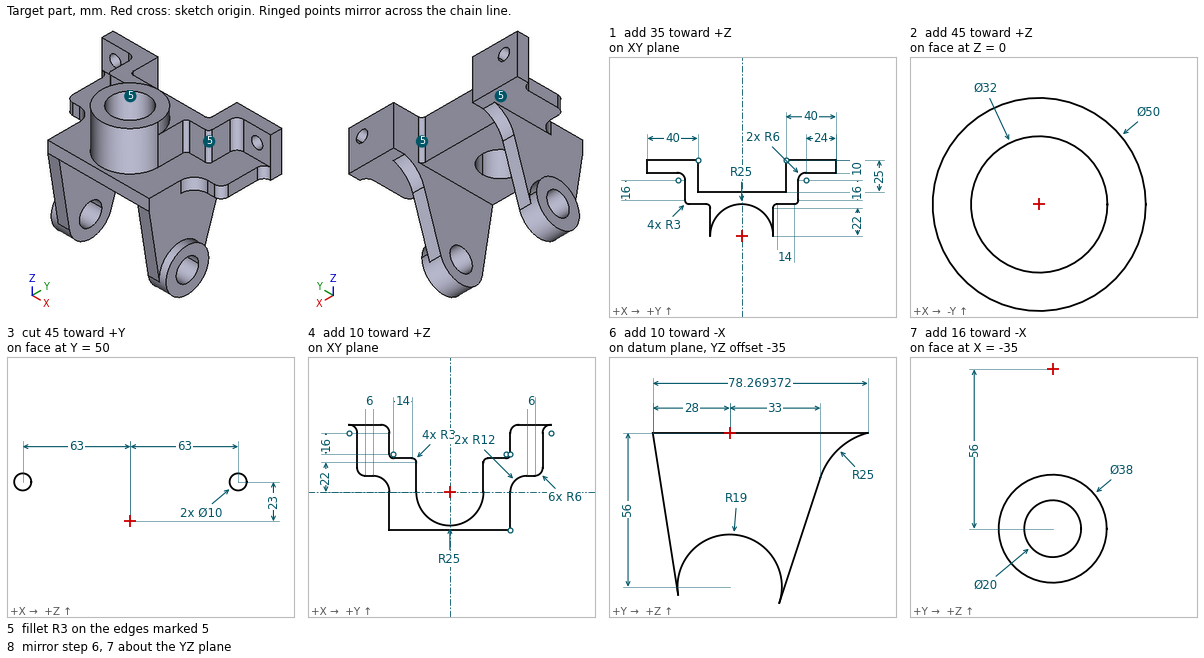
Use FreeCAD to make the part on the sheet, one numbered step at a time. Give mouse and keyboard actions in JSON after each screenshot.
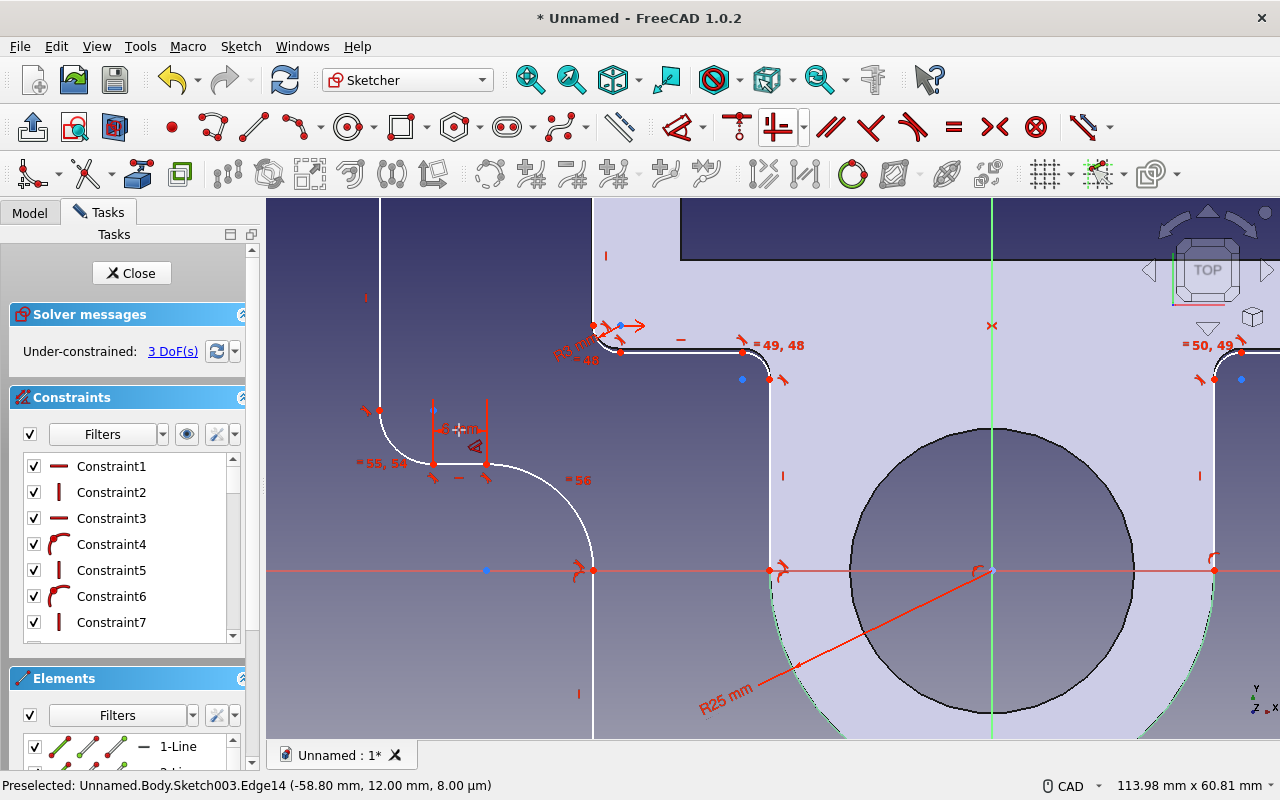
{"action": "left_click", "coordinate": [593, 227]}
{"action": "left_click", "coordinate": [559, 276]}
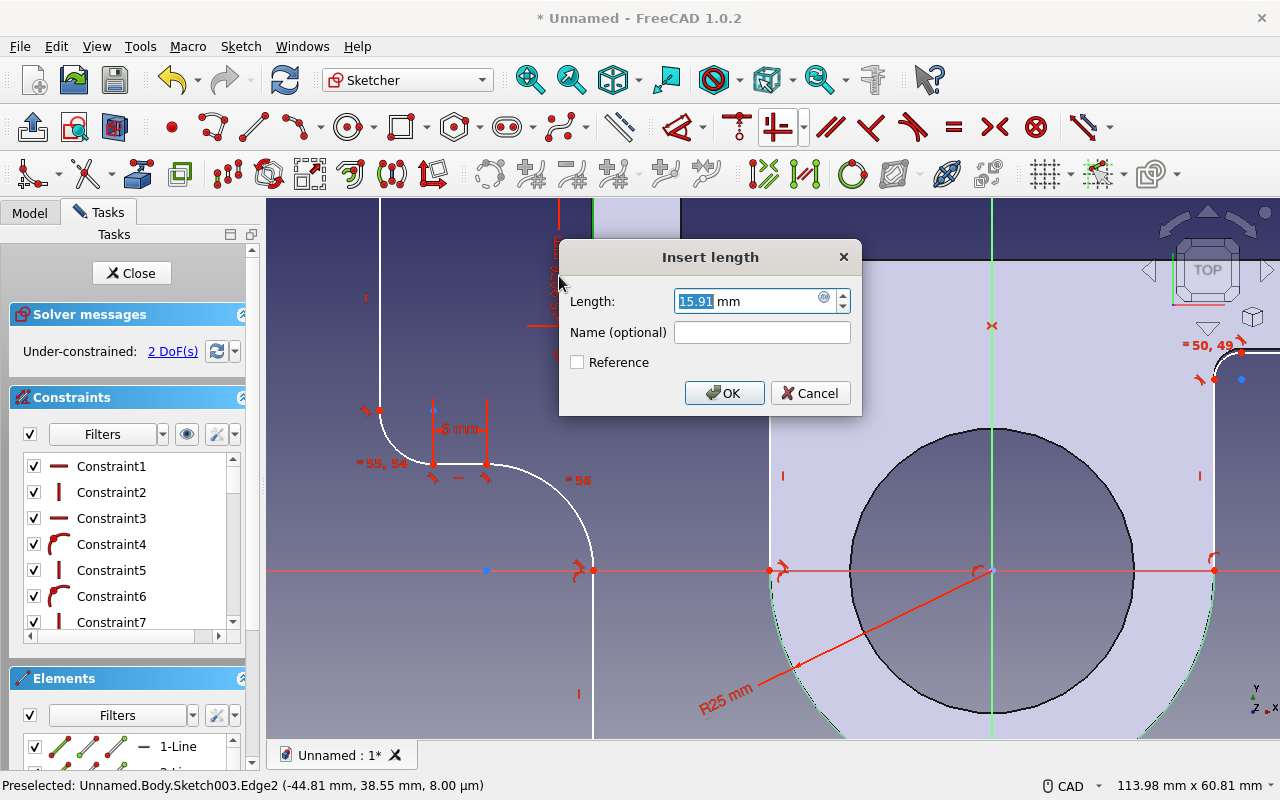
{"action": "type", "text": "16"}
{"action": "key", "text": "Return"}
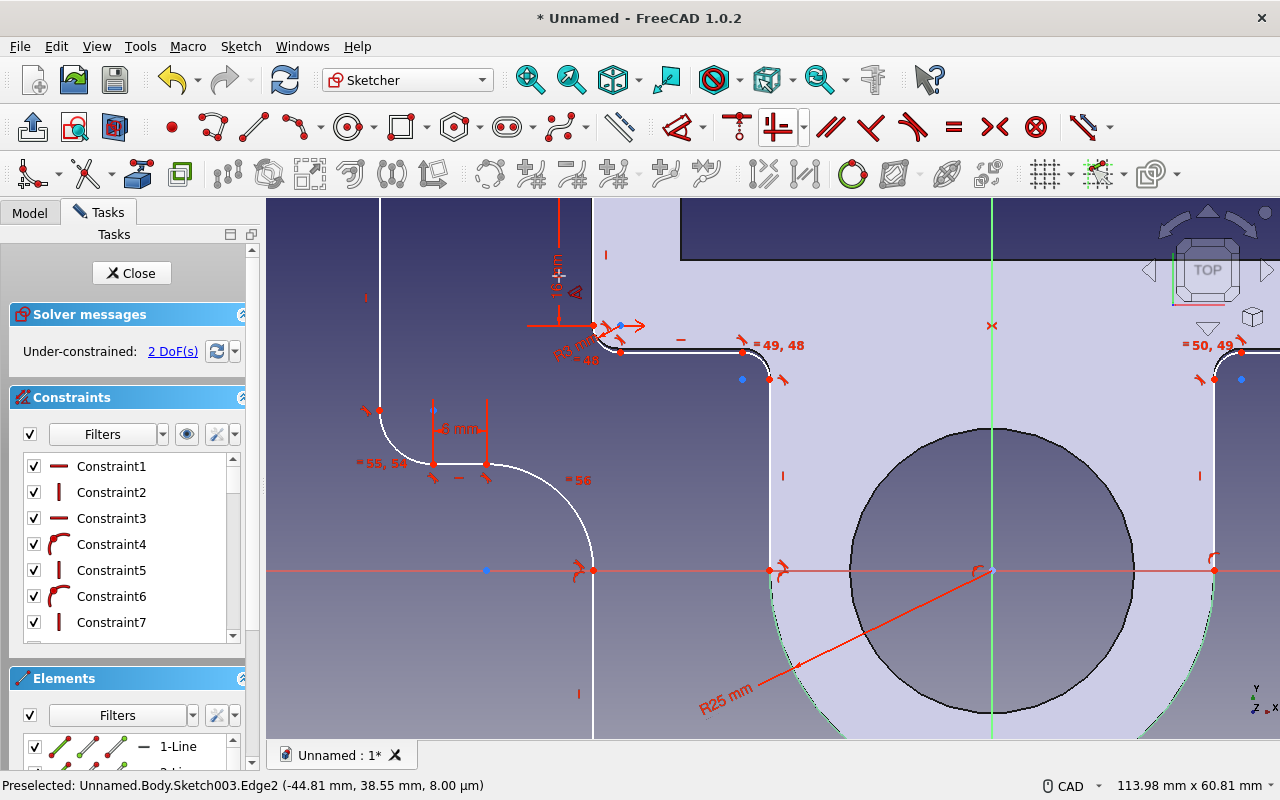
{"action": "left_click", "coordinate": [657, 353]}
{"action": "left_click", "coordinate": [682, 319]}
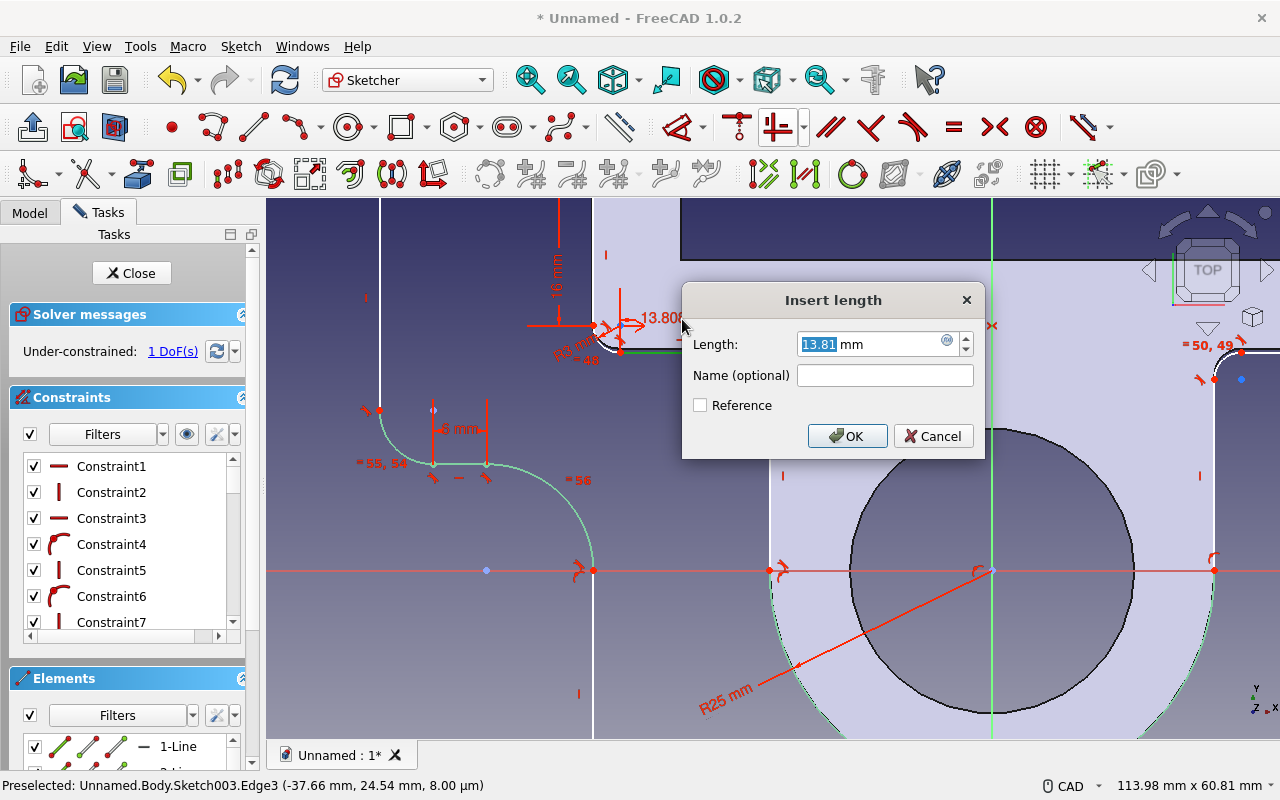
{"action": "type", "text": "14"}
{"action": "key", "text": "Return"}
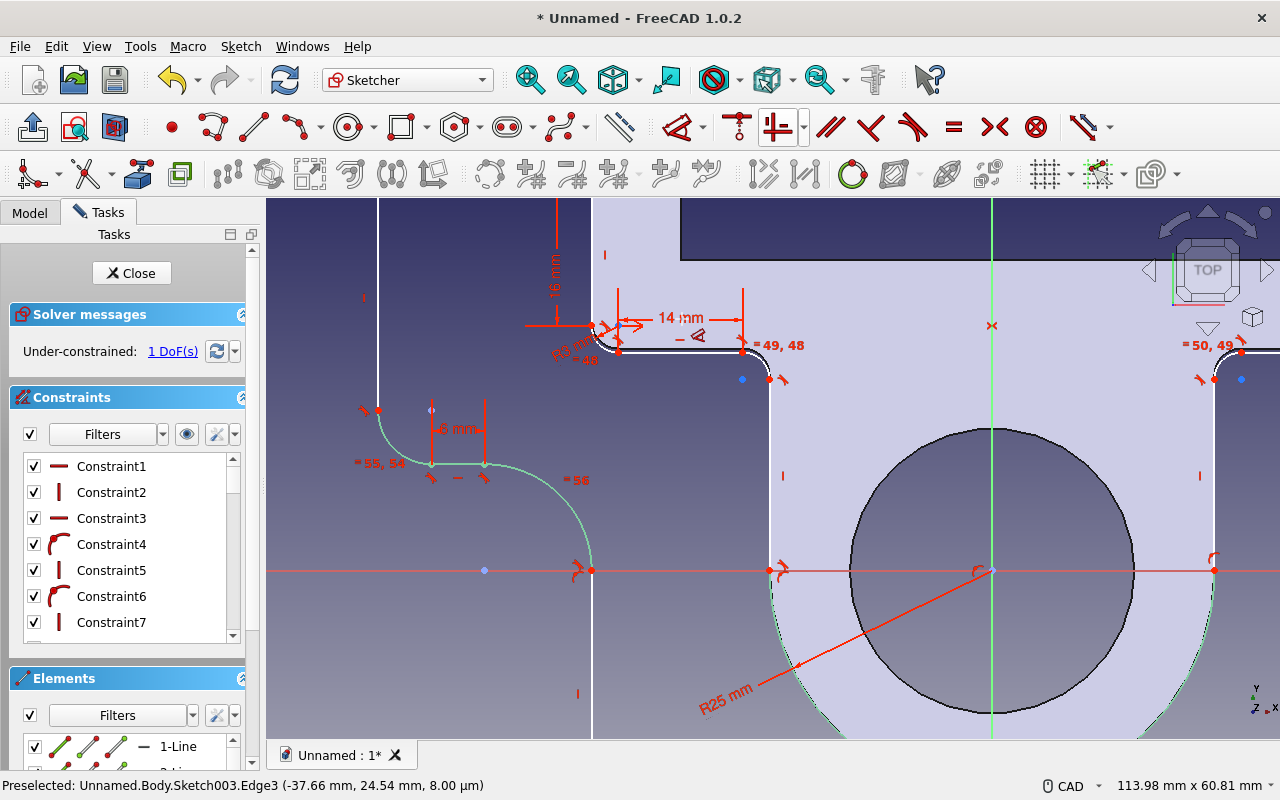
{"action": "left_click", "coordinate": [770, 437]}
{"action": "left_click", "coordinate": [736, 475]}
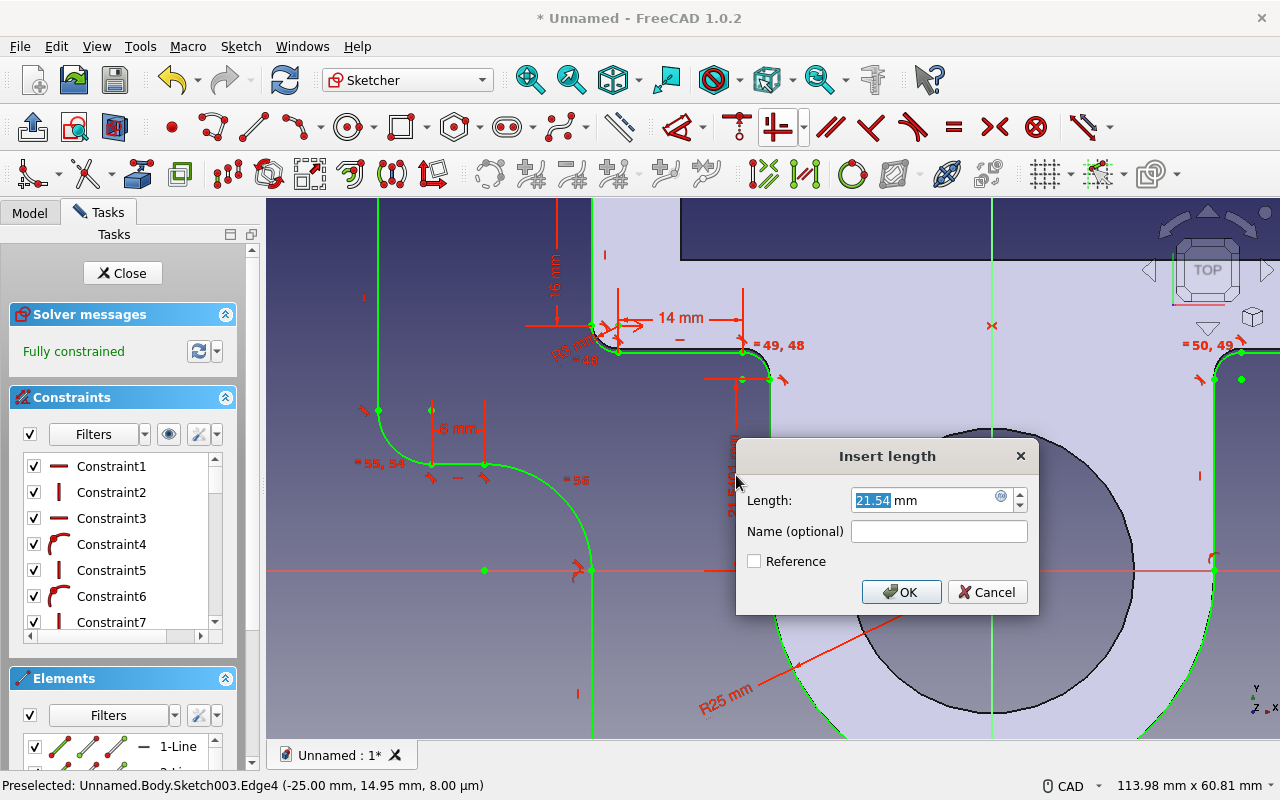
{"action": "type", "text": "22"}
{"action": "key", "text": "Return"}
{"action": "key", "text": "Escape"}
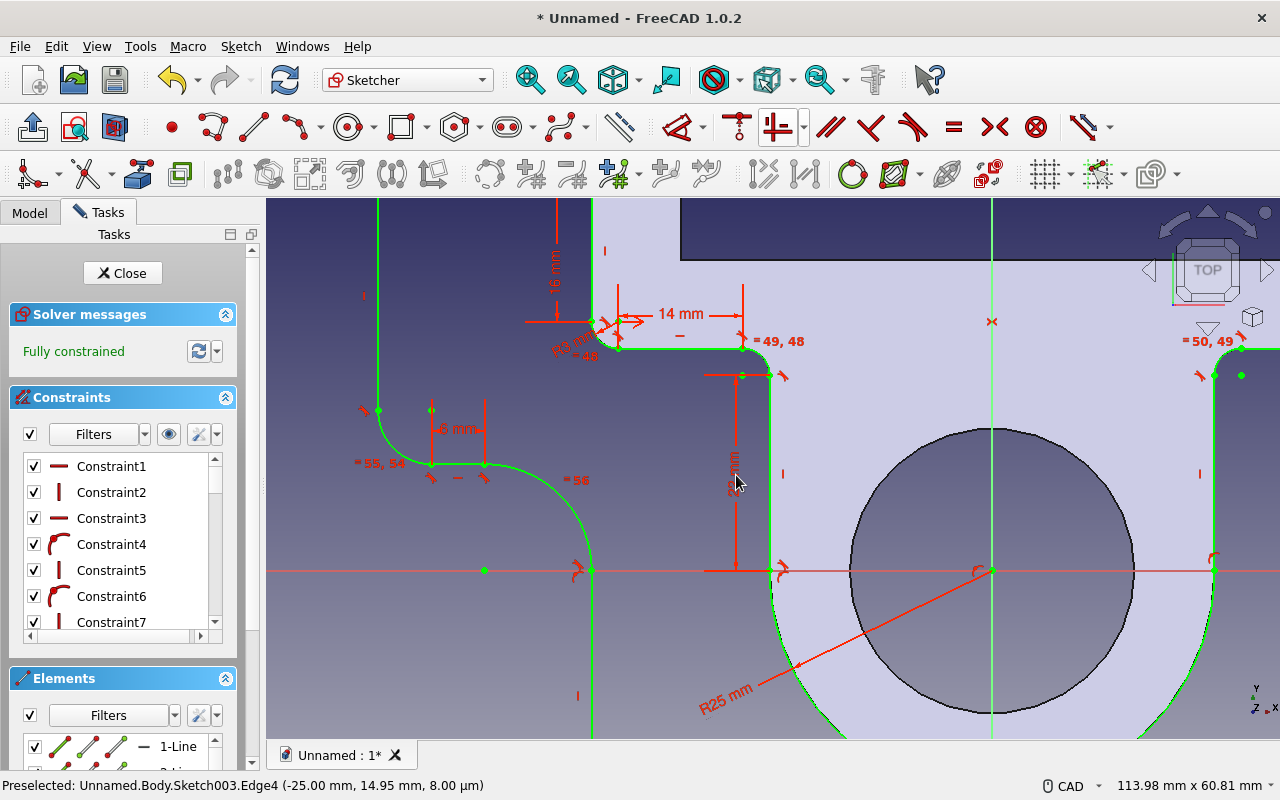
{"action": "left_click", "coordinate": [123, 273]}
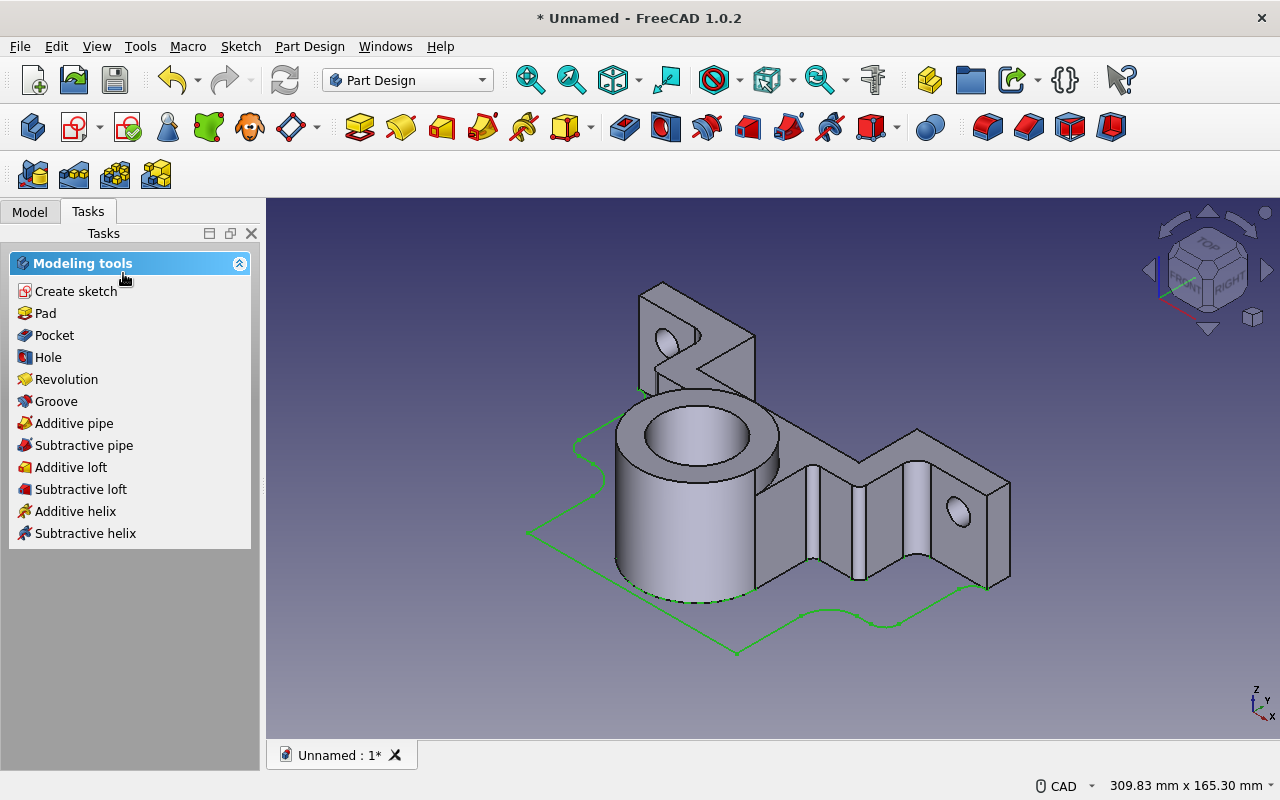
{"action": "left_click", "coordinate": [360, 128]}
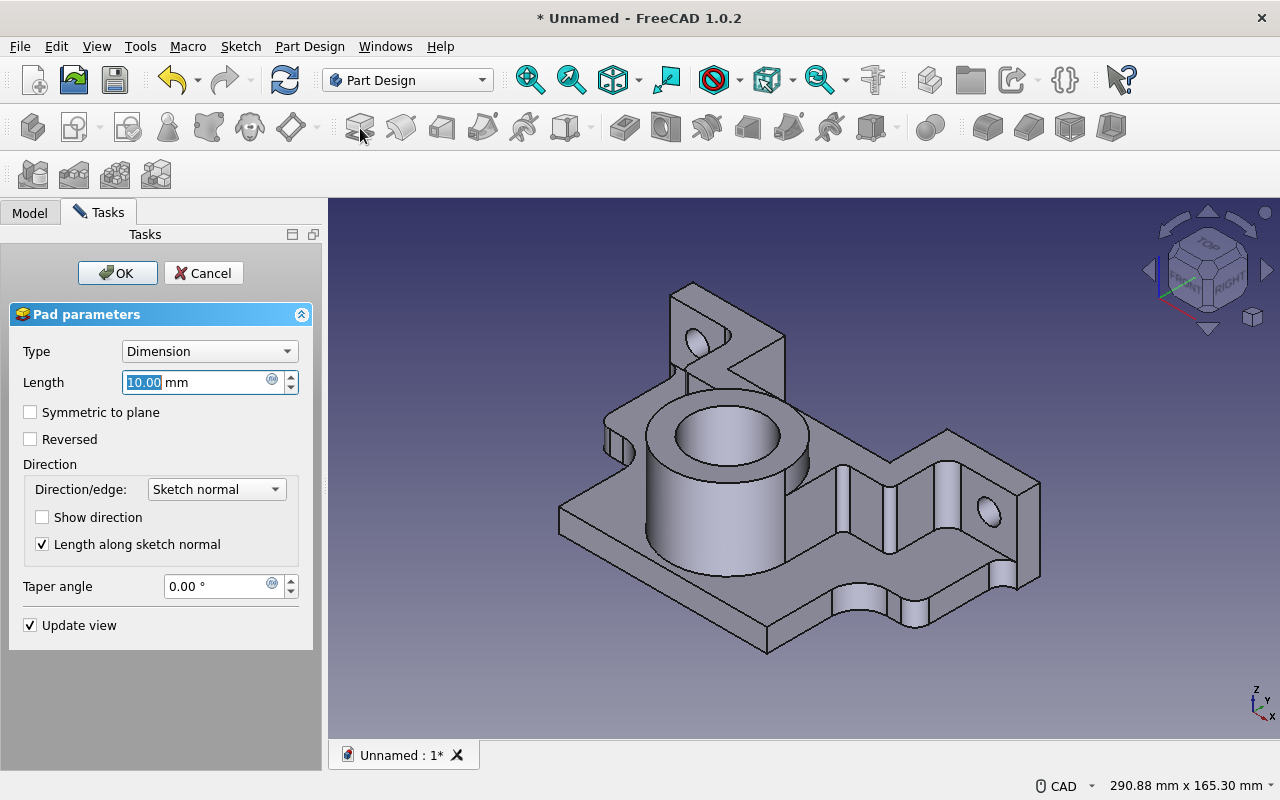
{"action": "type", "text": "10"}
{"action": "key", "text": "Tab"}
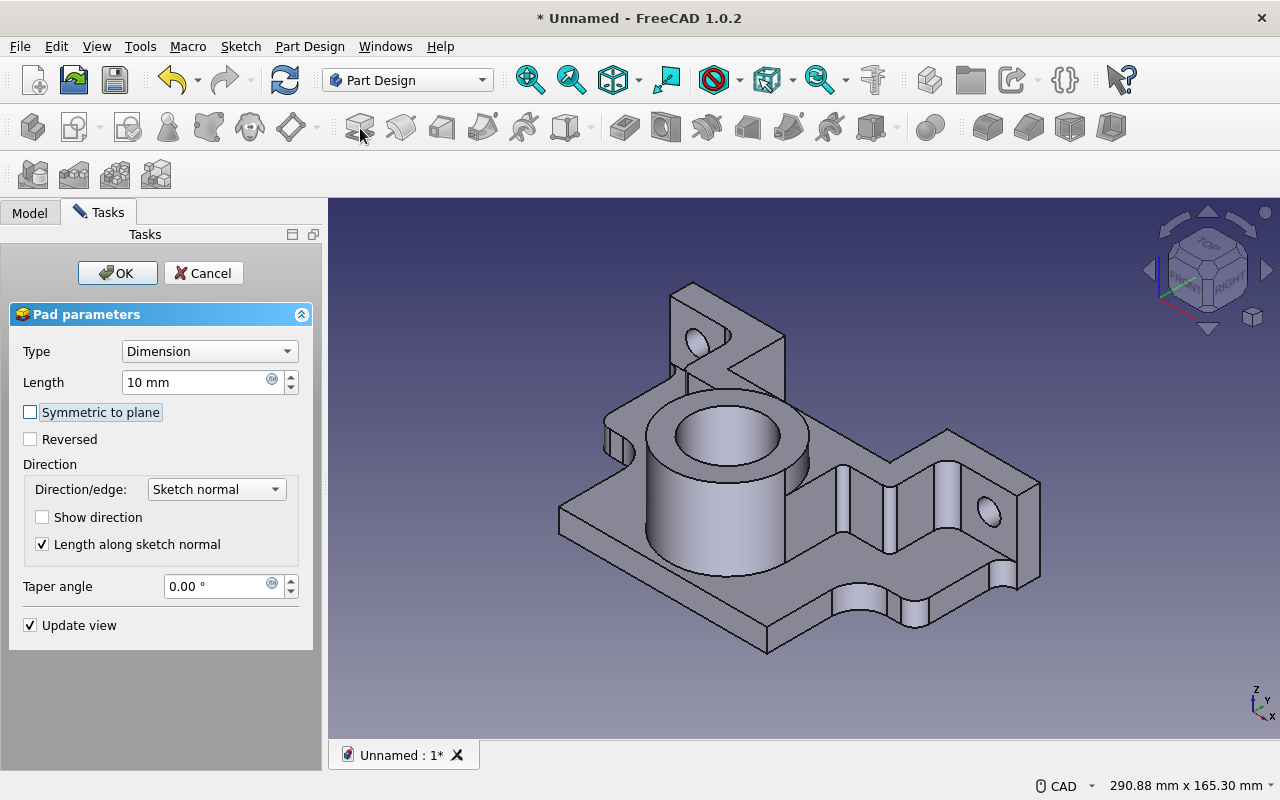
{"action": "left_click", "coordinate": [118, 273]}